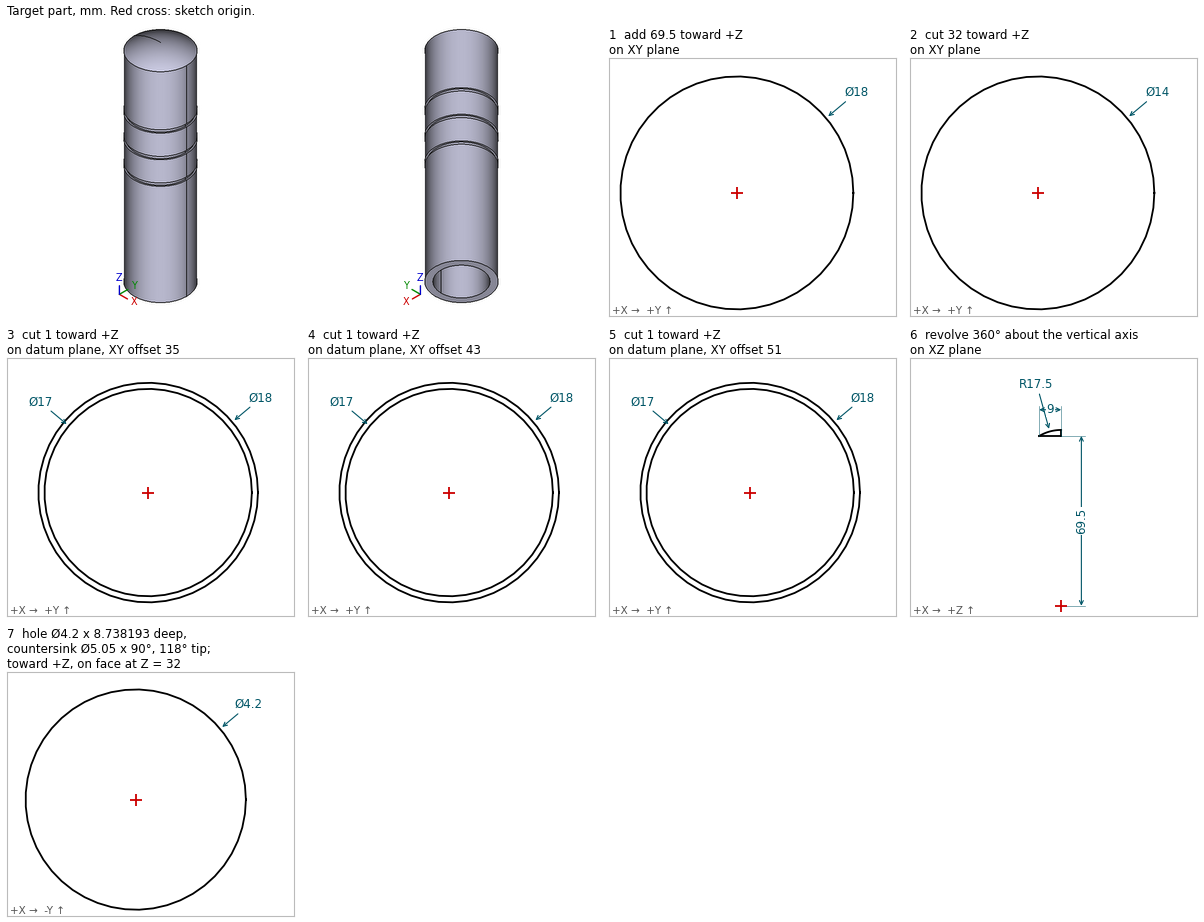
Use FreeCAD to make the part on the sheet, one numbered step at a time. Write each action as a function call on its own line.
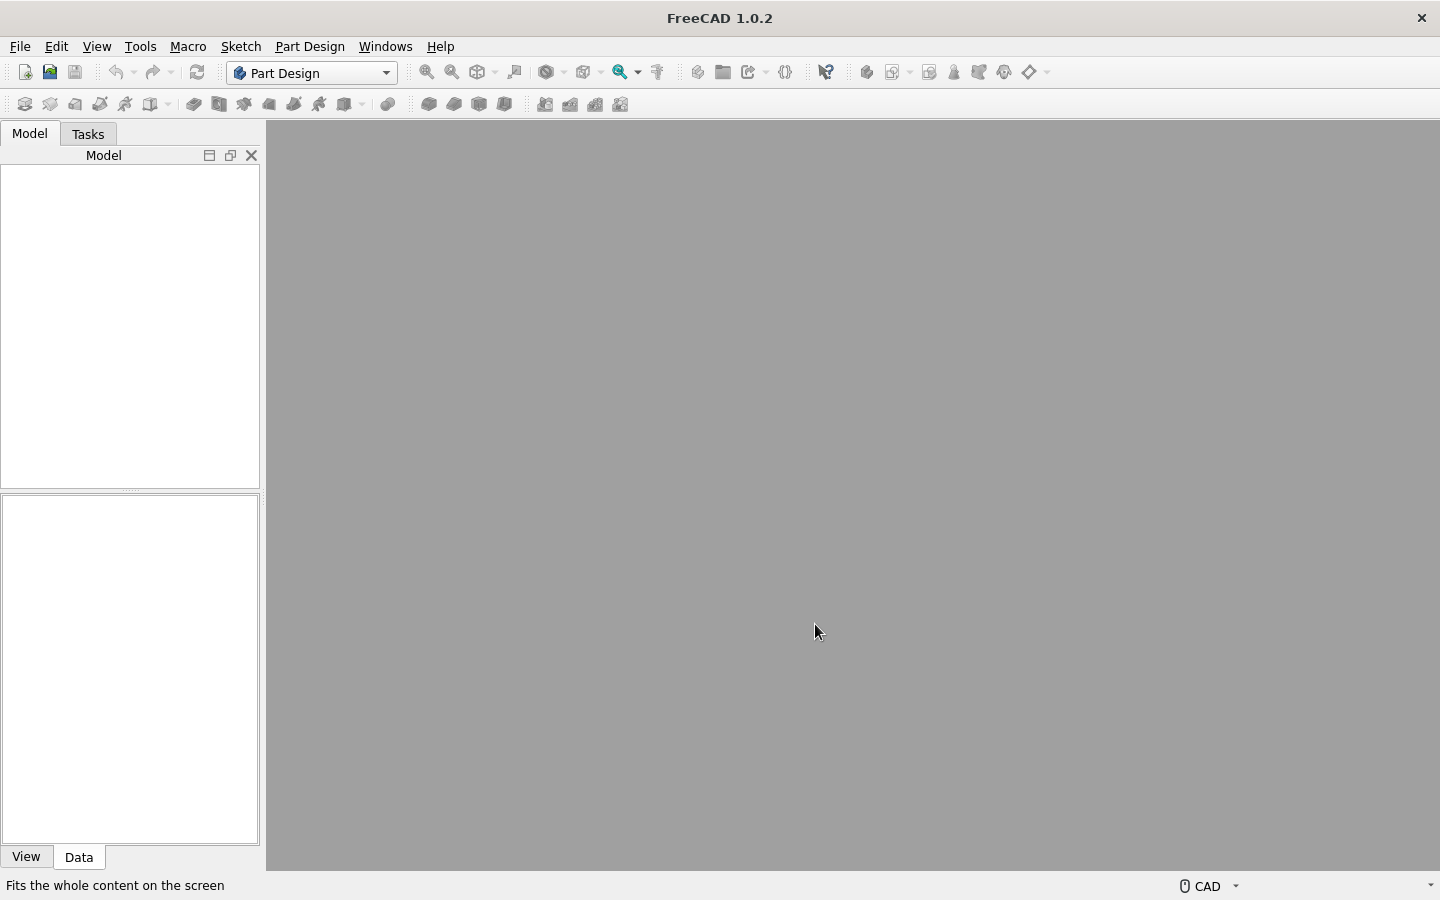
click(25, 72)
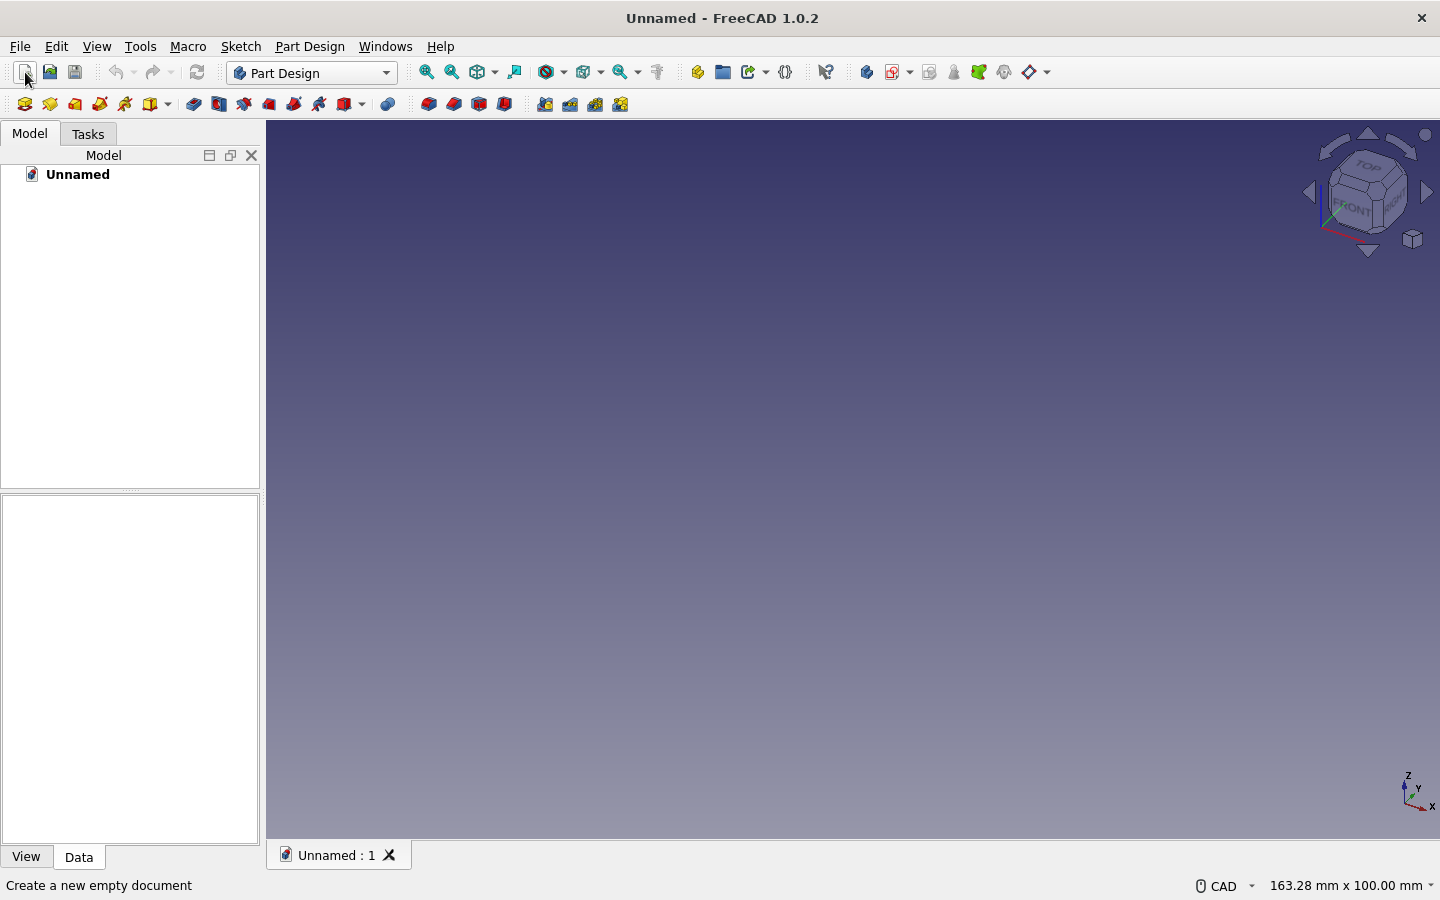
click(892, 72)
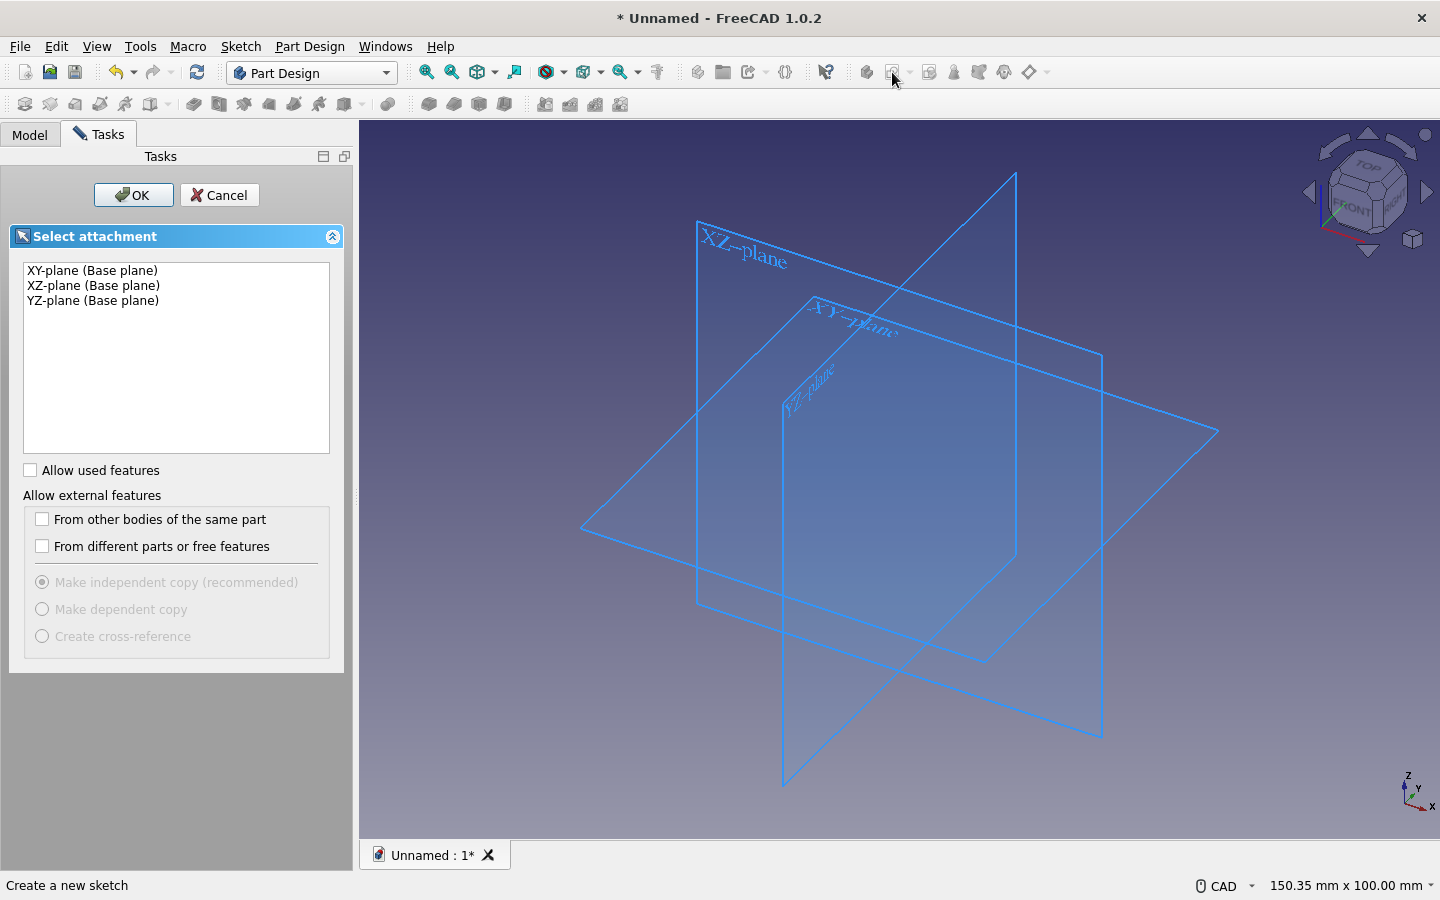
click(84, 270)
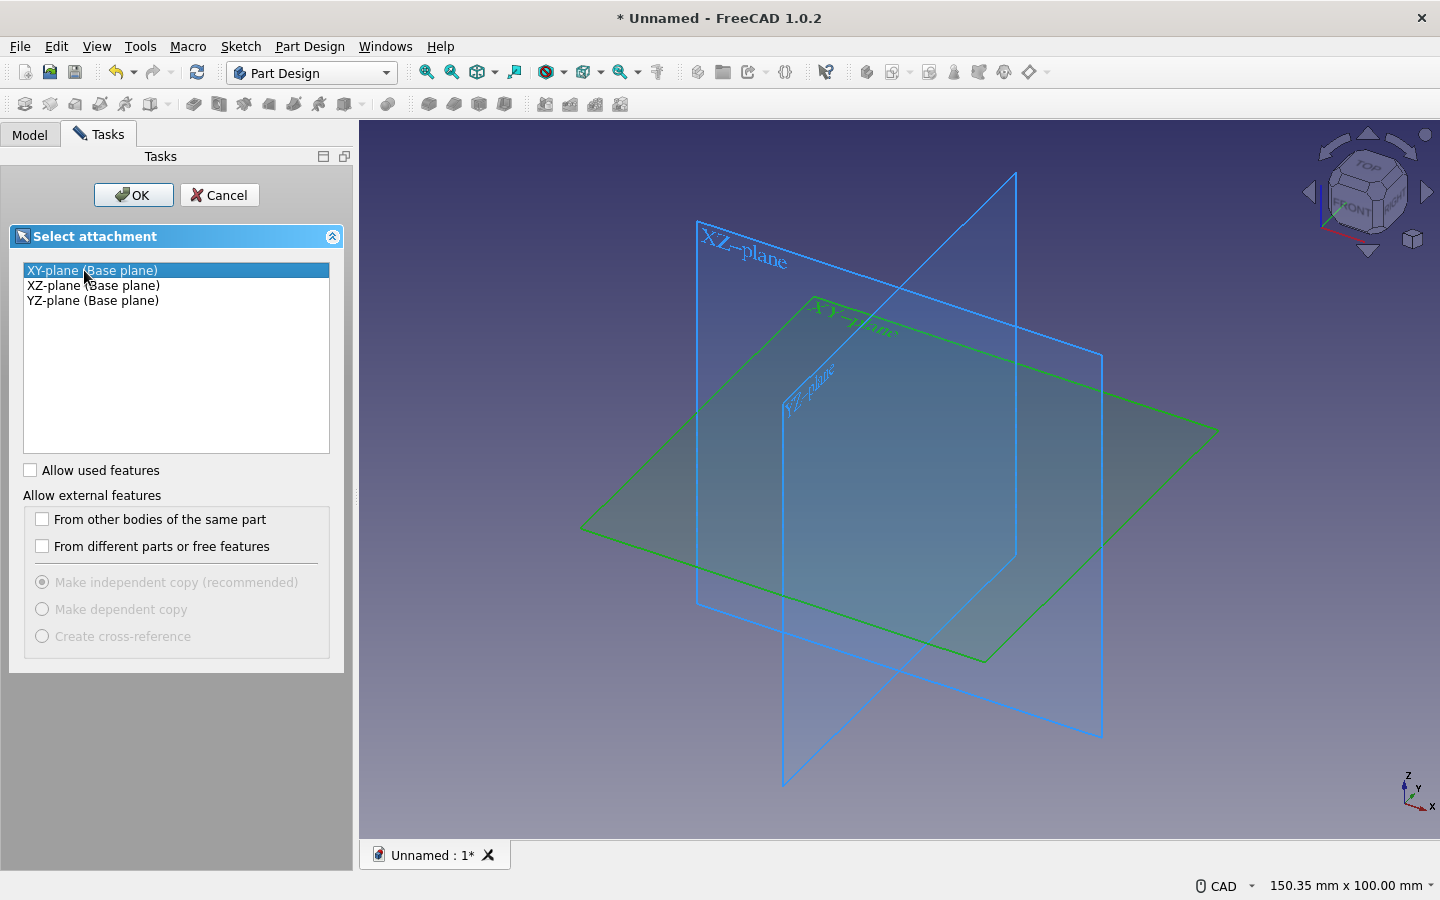
click(134, 195)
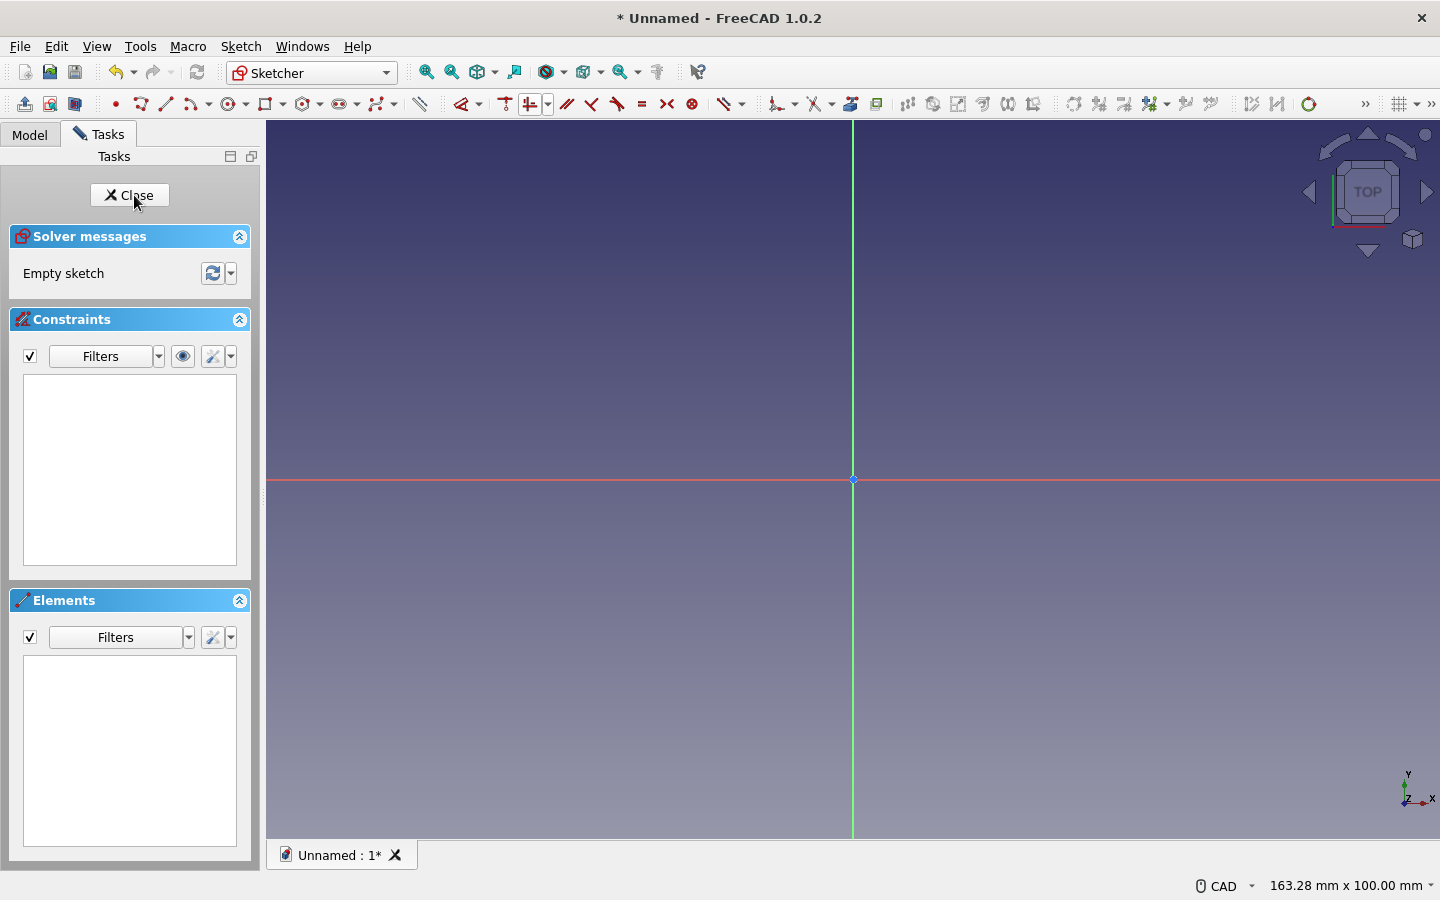
scroll(883, 480, up, 6)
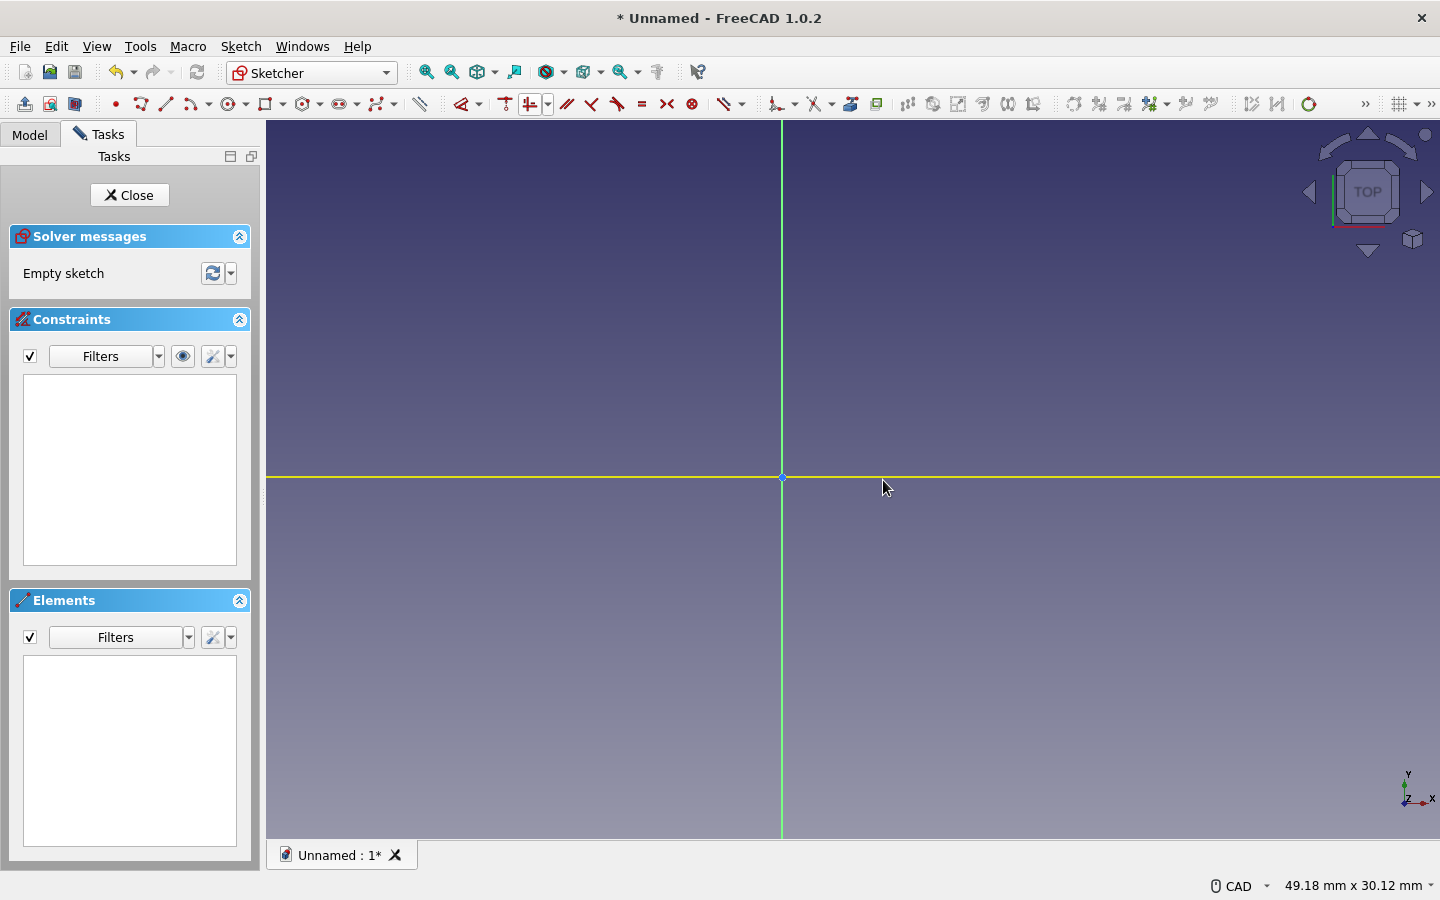
key(g)
key(c)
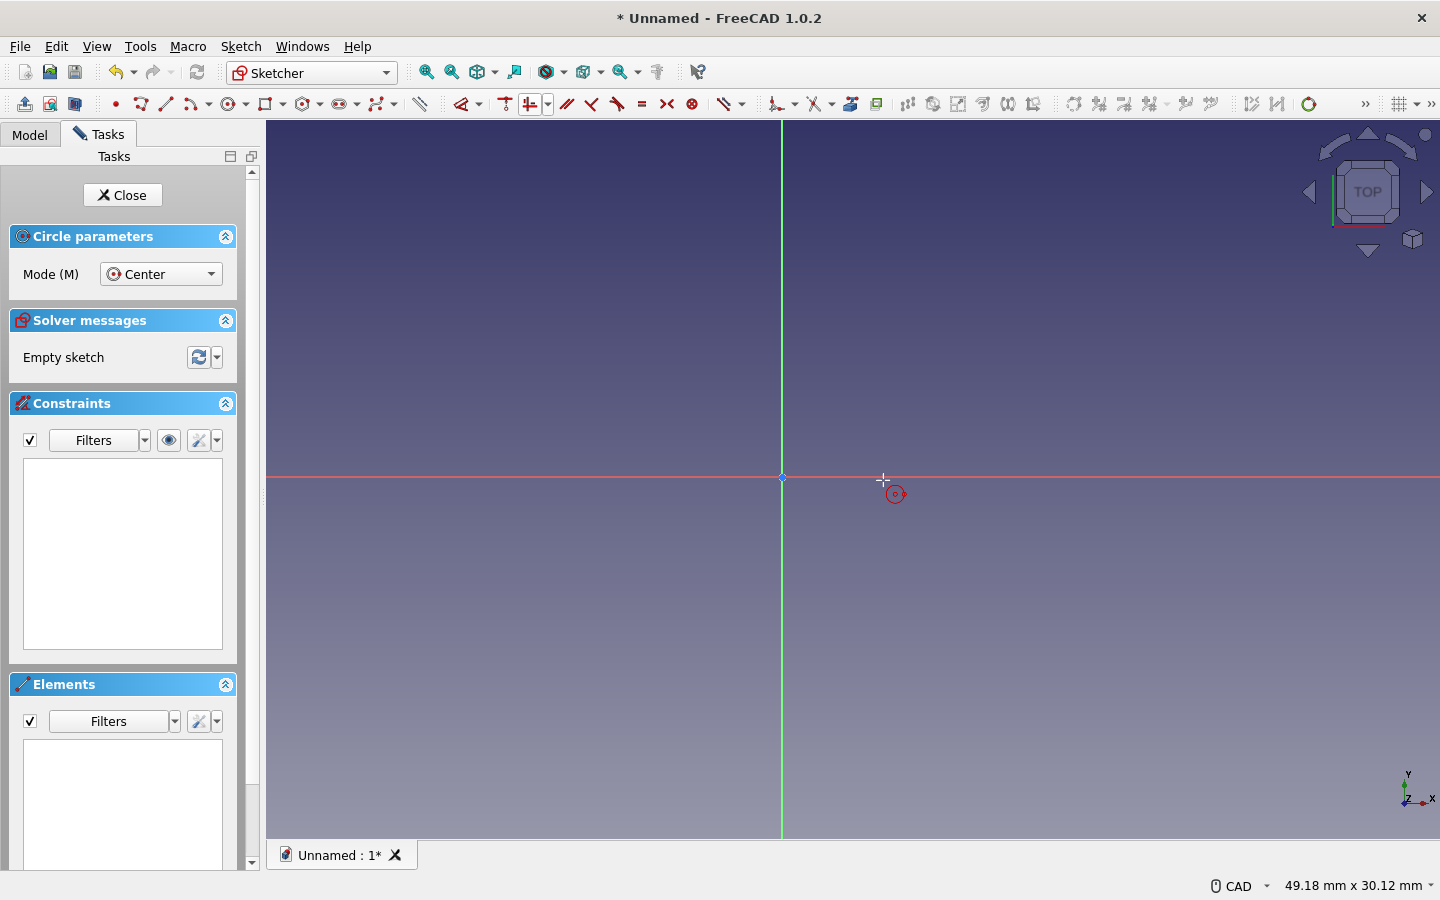
click(782, 477)
click(934, 325)
key(Escape)